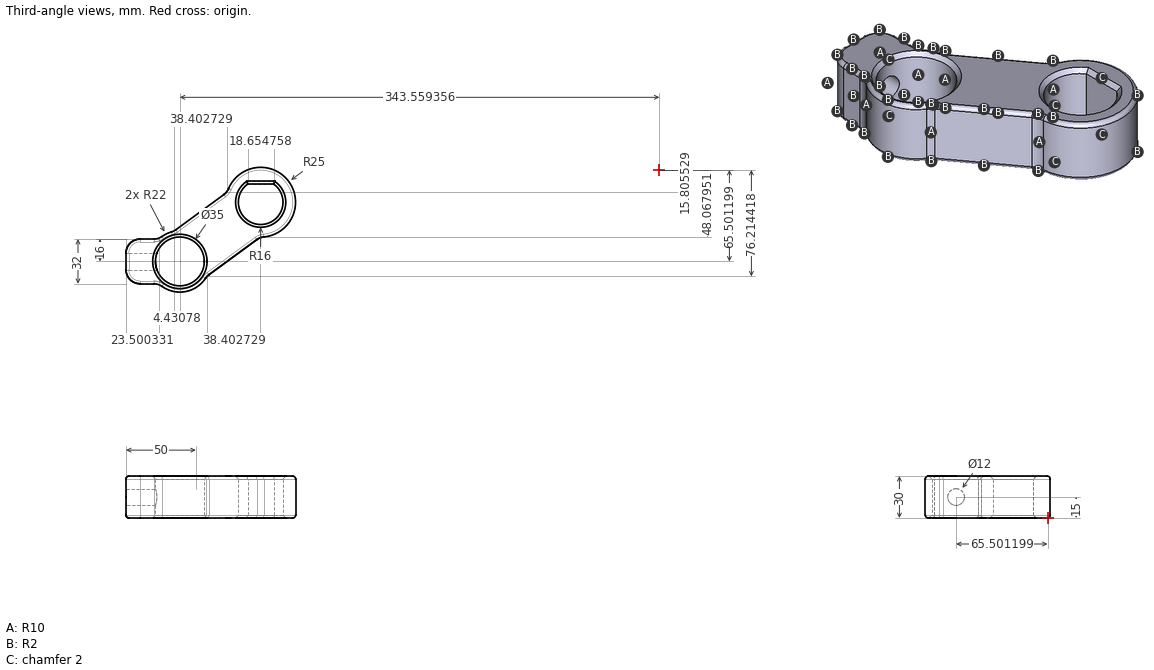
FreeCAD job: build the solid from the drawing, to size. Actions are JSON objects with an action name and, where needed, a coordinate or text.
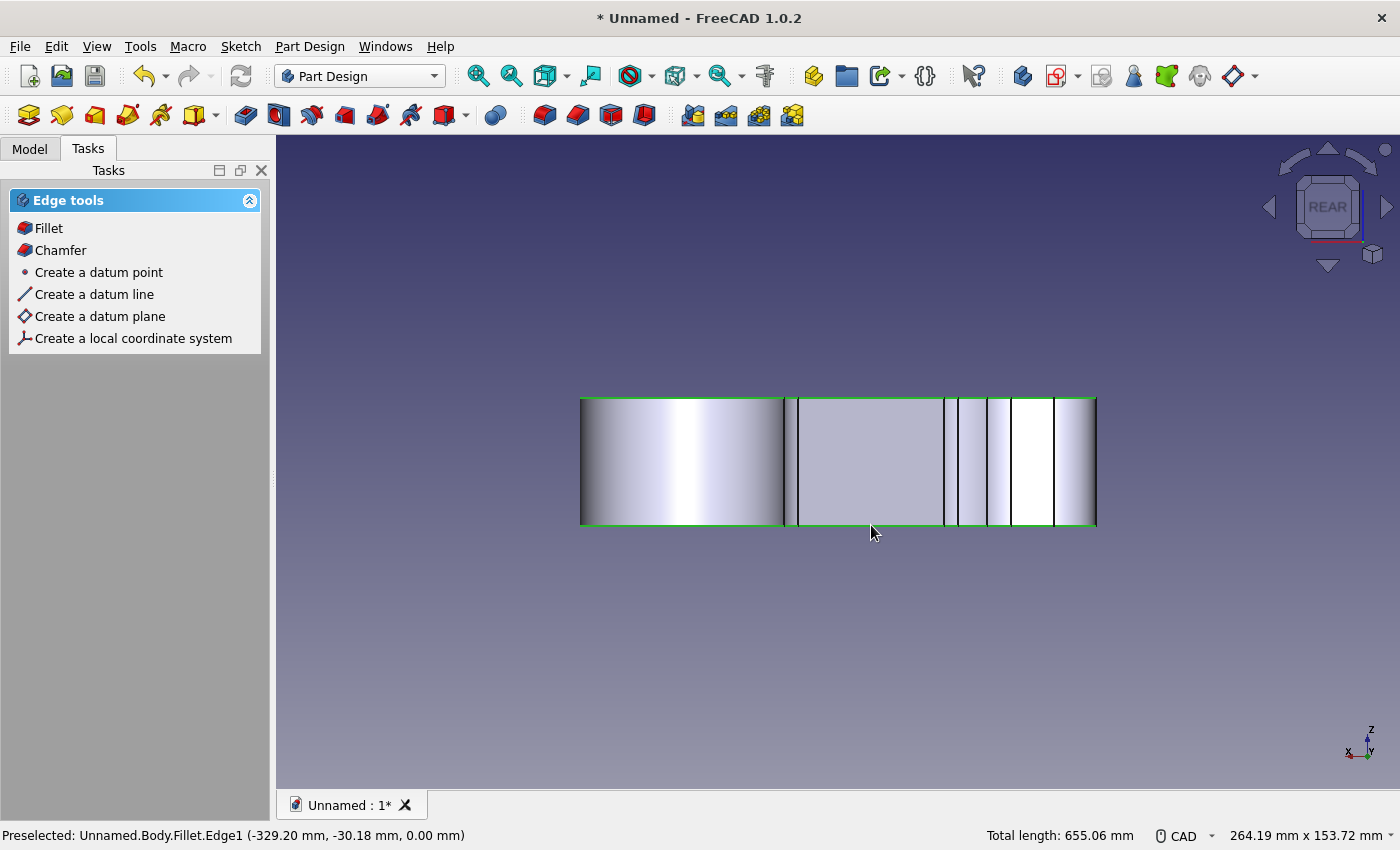
{"action": "left_click", "coordinate": [545, 116]}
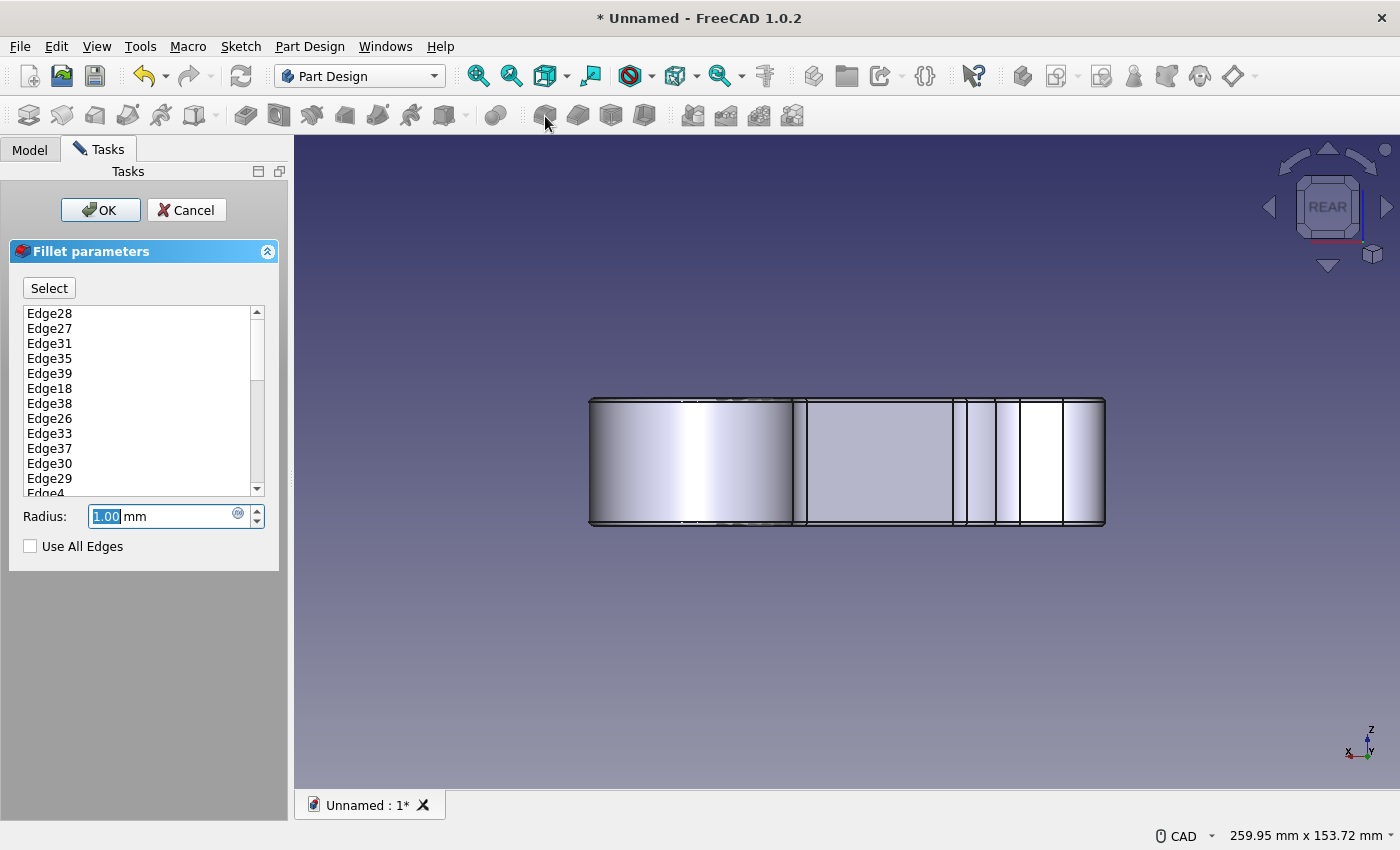
{"action": "type", "text": "2"}
{"action": "key", "text": "Tab"}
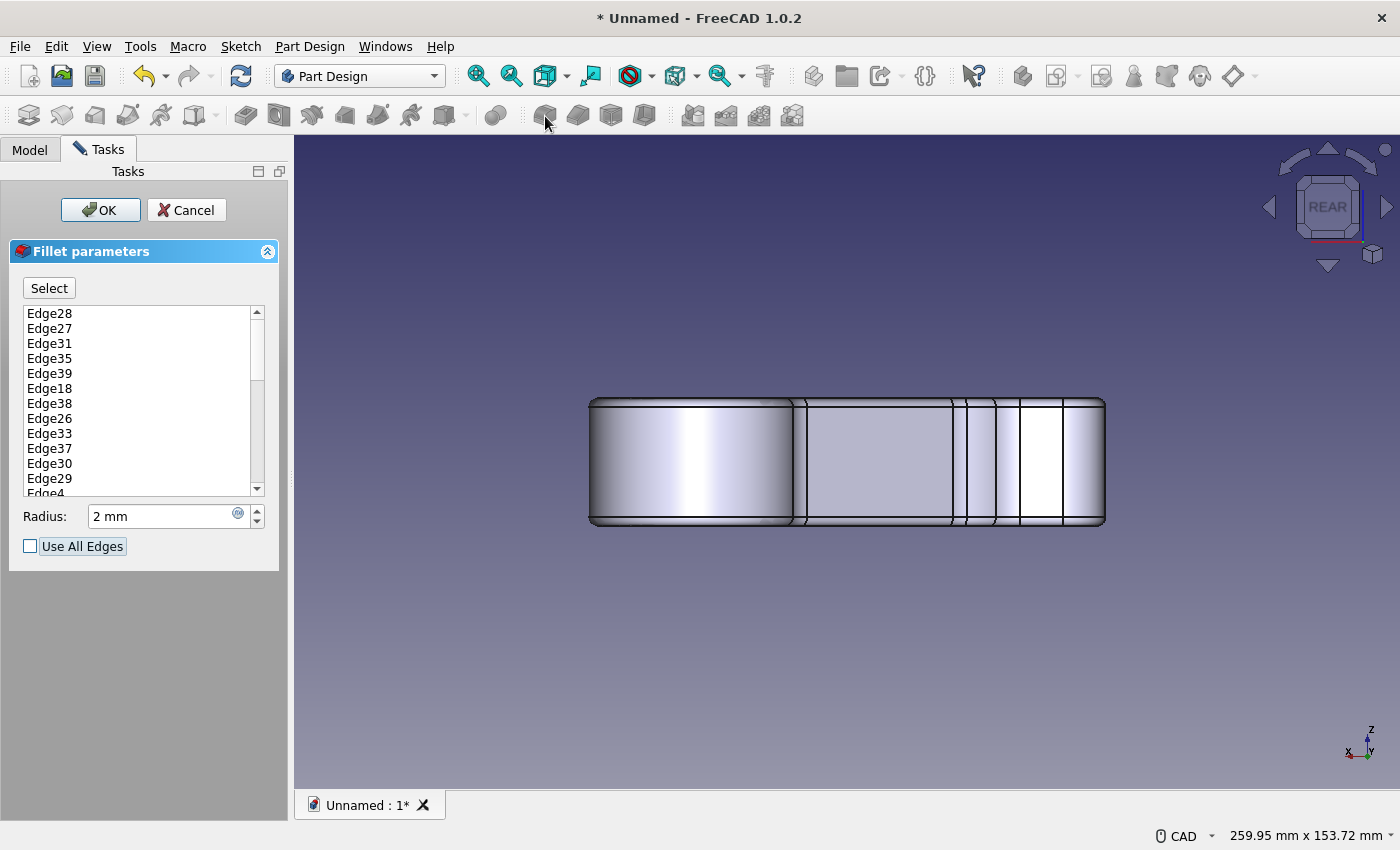
{"action": "left_click", "coordinate": [101, 210]}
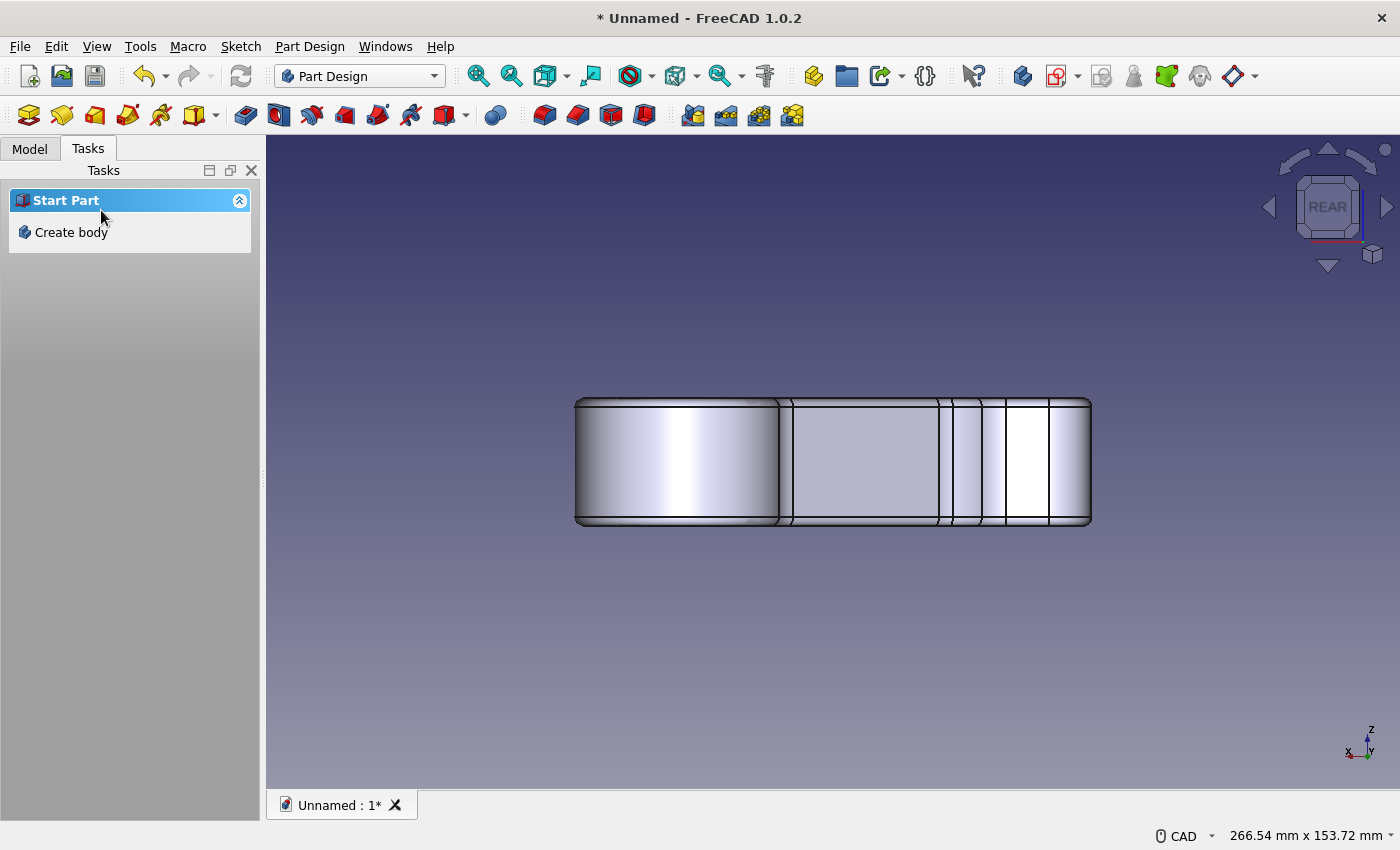
{"action": "key", "text": "0"}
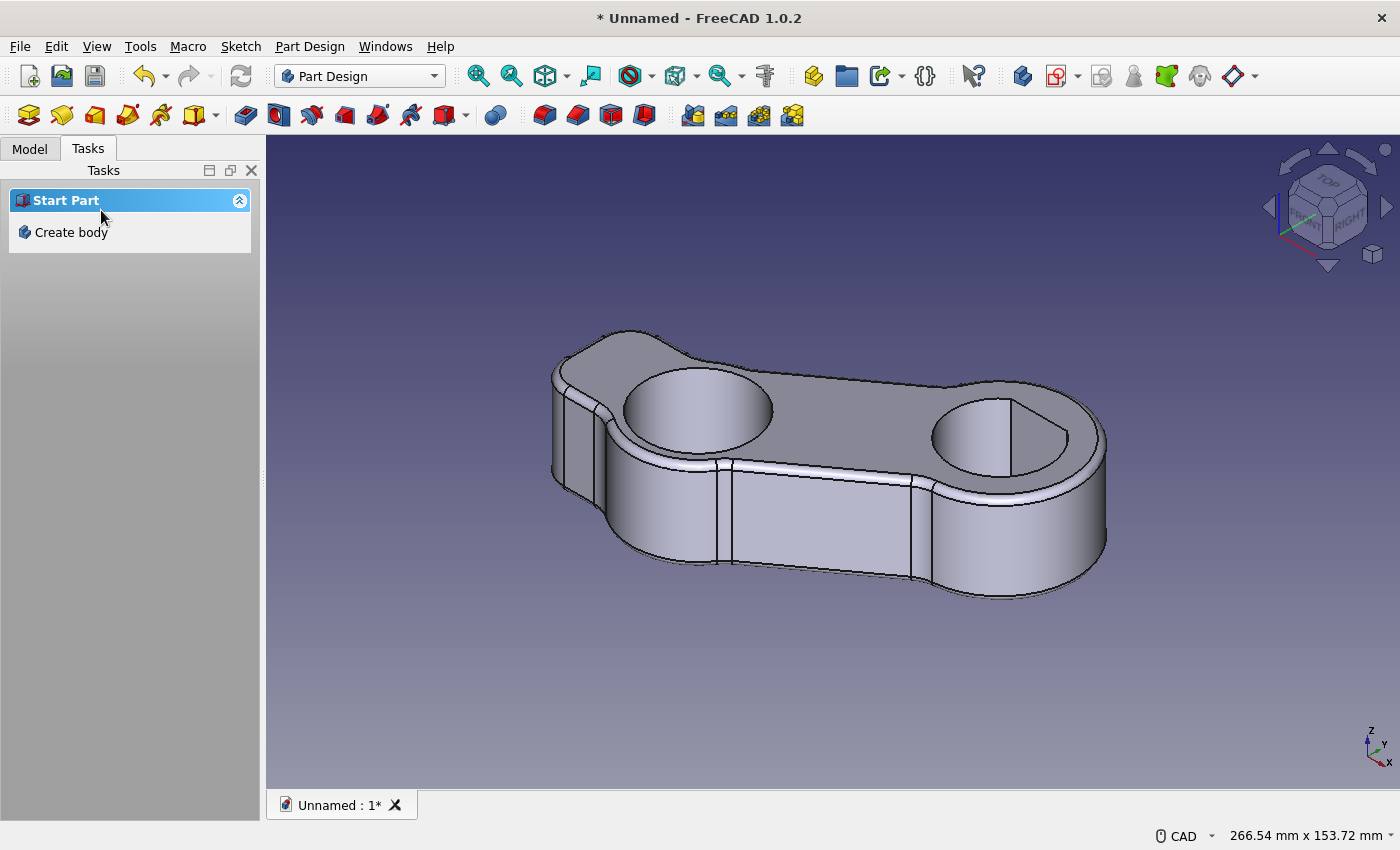
{"action": "left_click", "coordinate": [934, 428]}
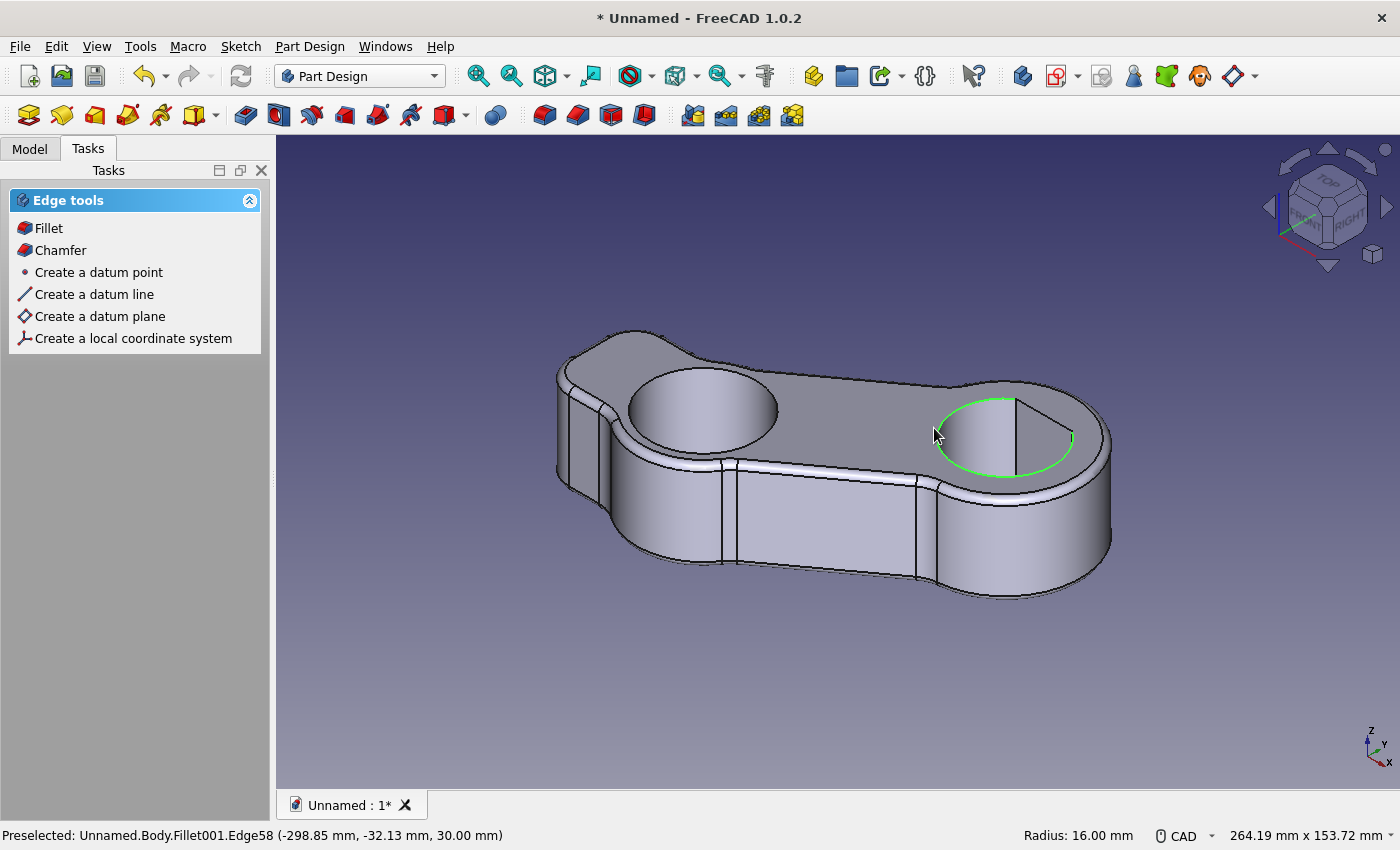
{"action": "left_click", "coordinate": [1044, 414], "text": "ctrl"}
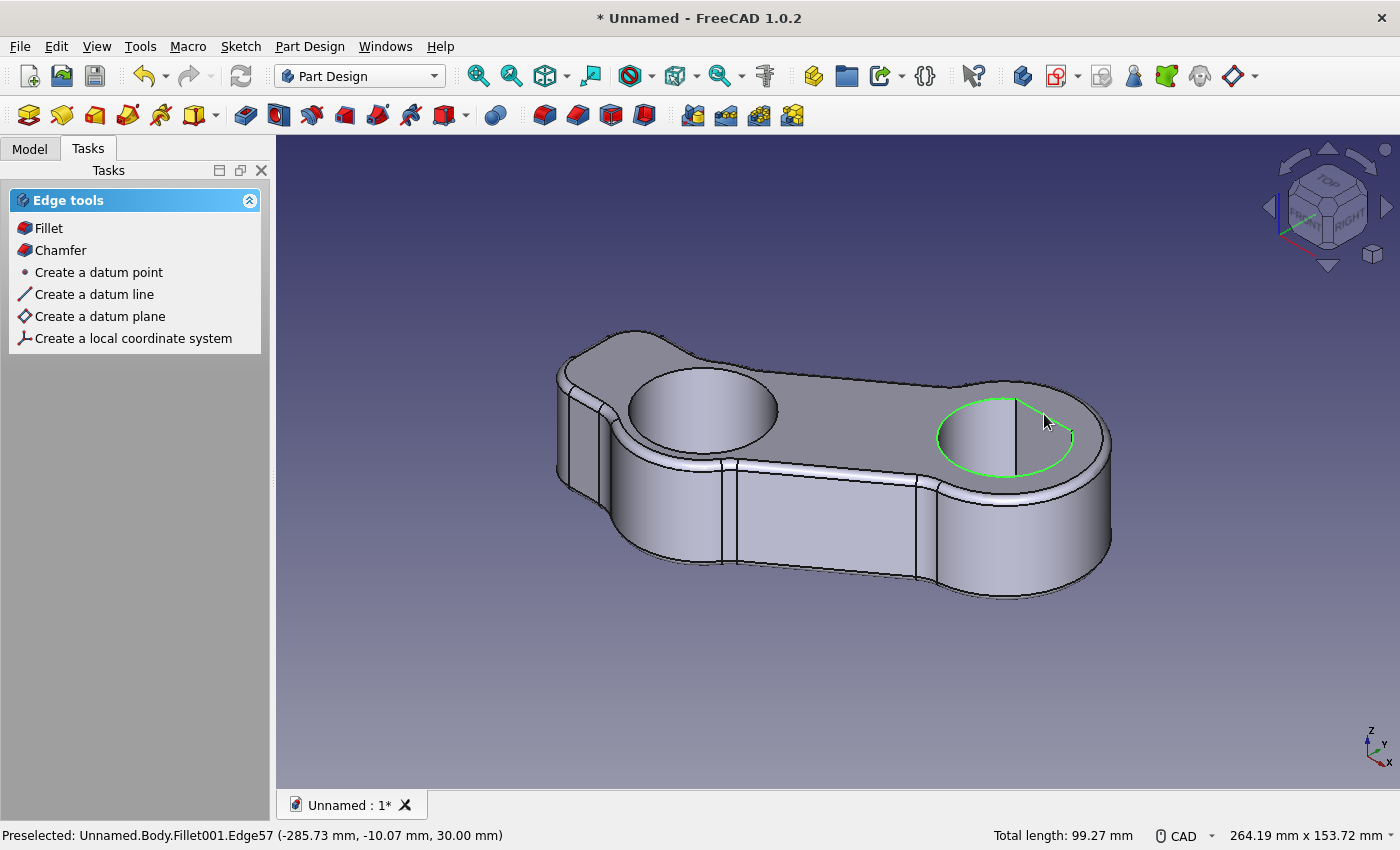
{"action": "left_click", "coordinate": [651, 379], "text": "ctrl"}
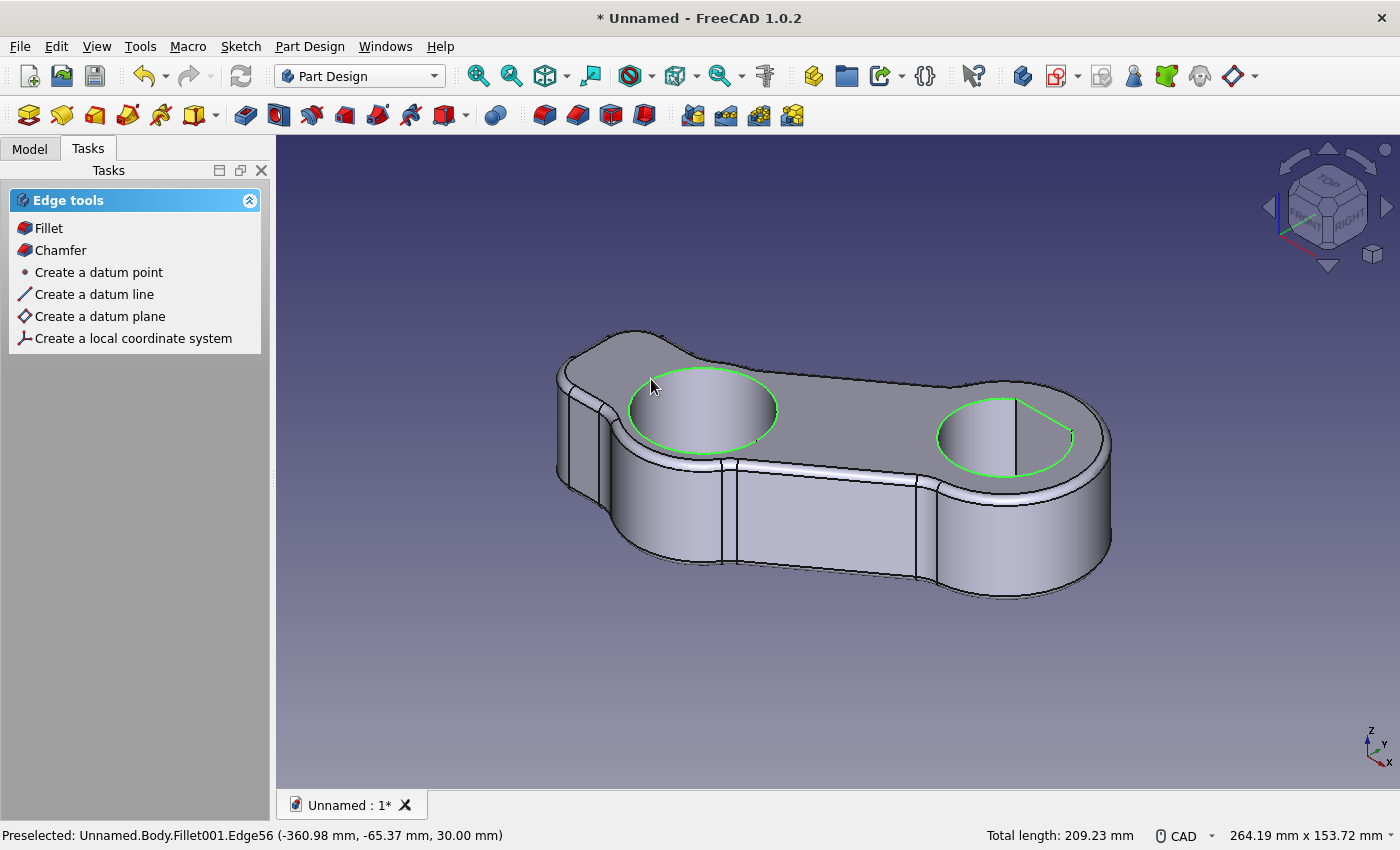
{"action": "key", "text": "2"}